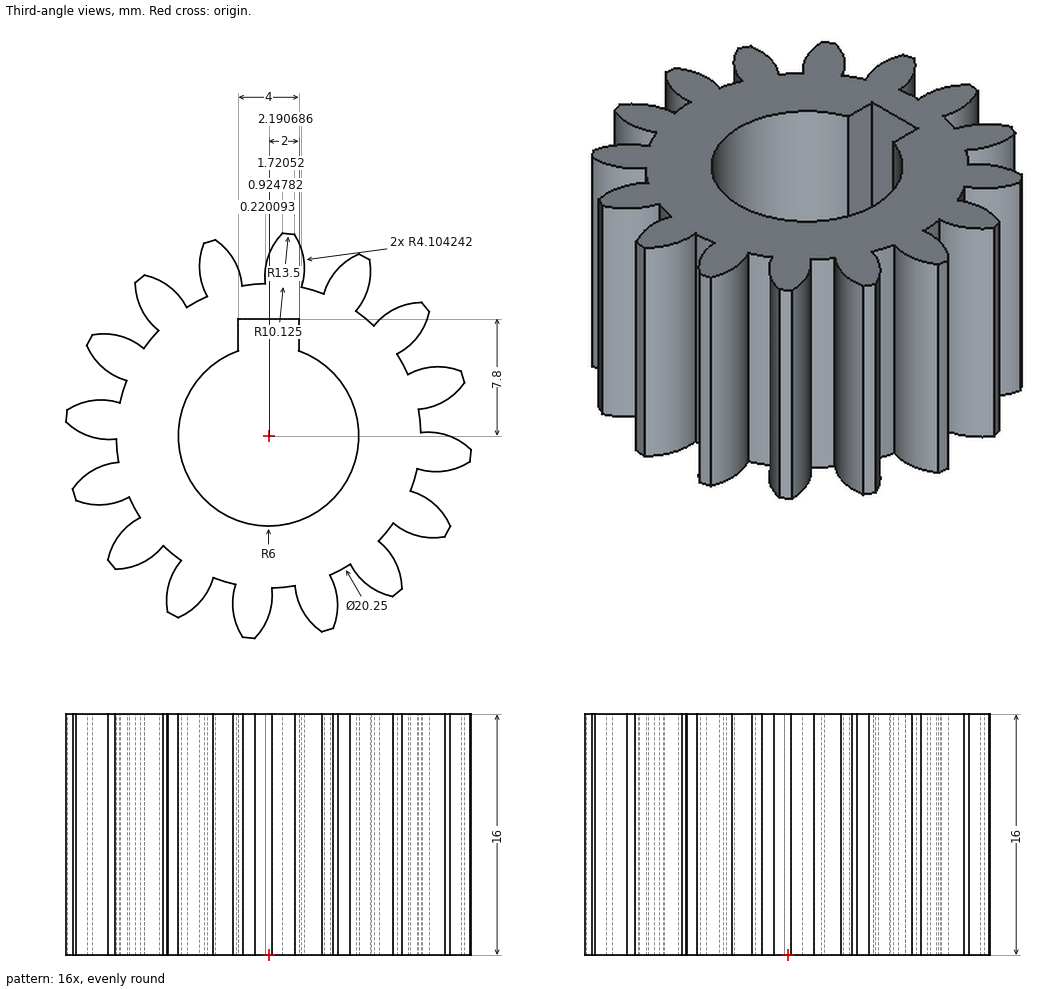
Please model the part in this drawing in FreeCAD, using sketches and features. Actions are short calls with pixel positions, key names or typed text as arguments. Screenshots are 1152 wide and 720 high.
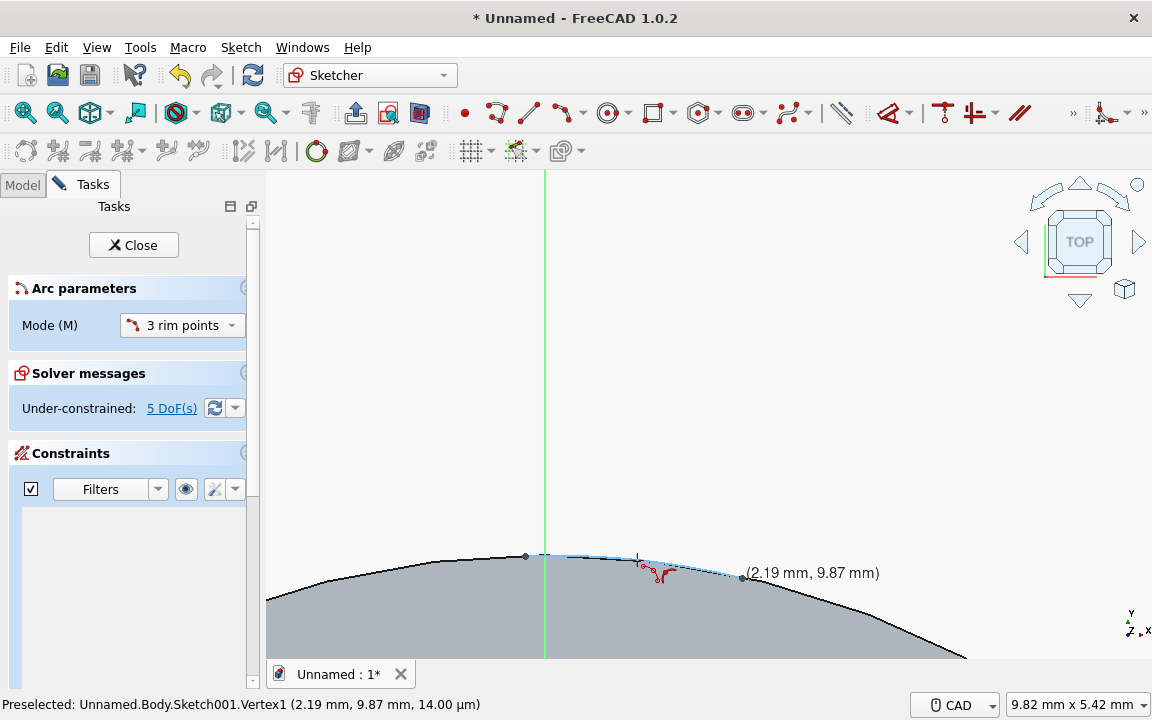
click(700, 261)
click(757, 414)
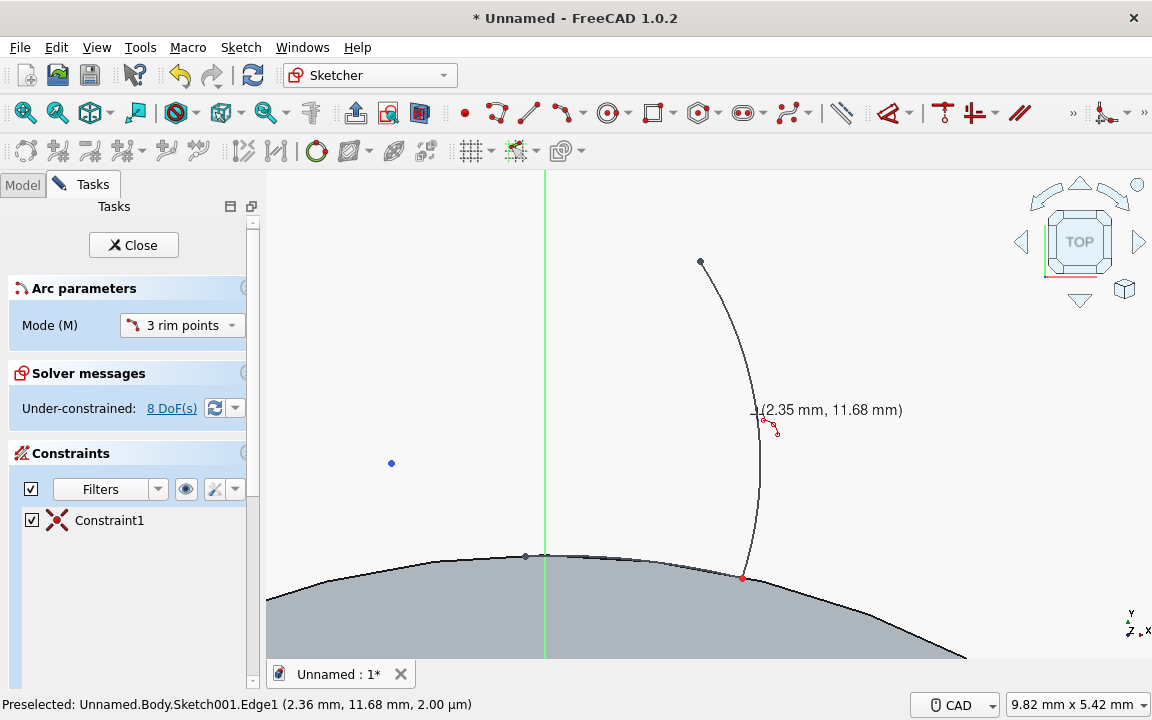
click(700, 262)
click(628, 254)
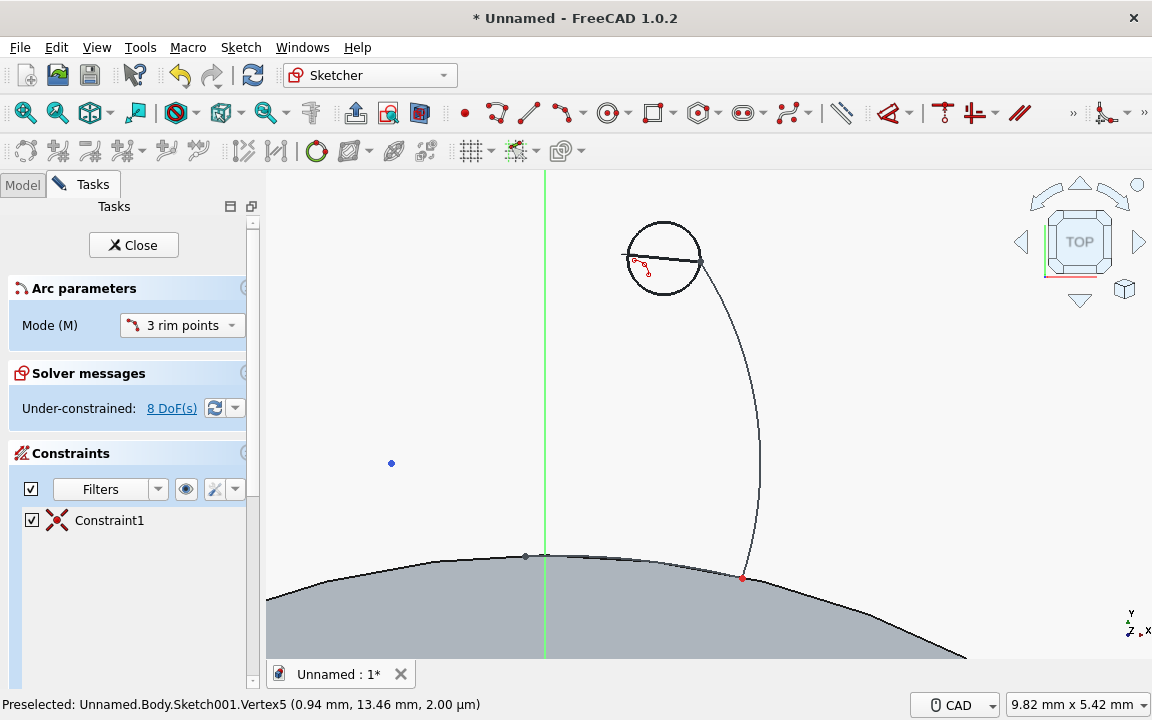
scroll(664, 257, up, 17)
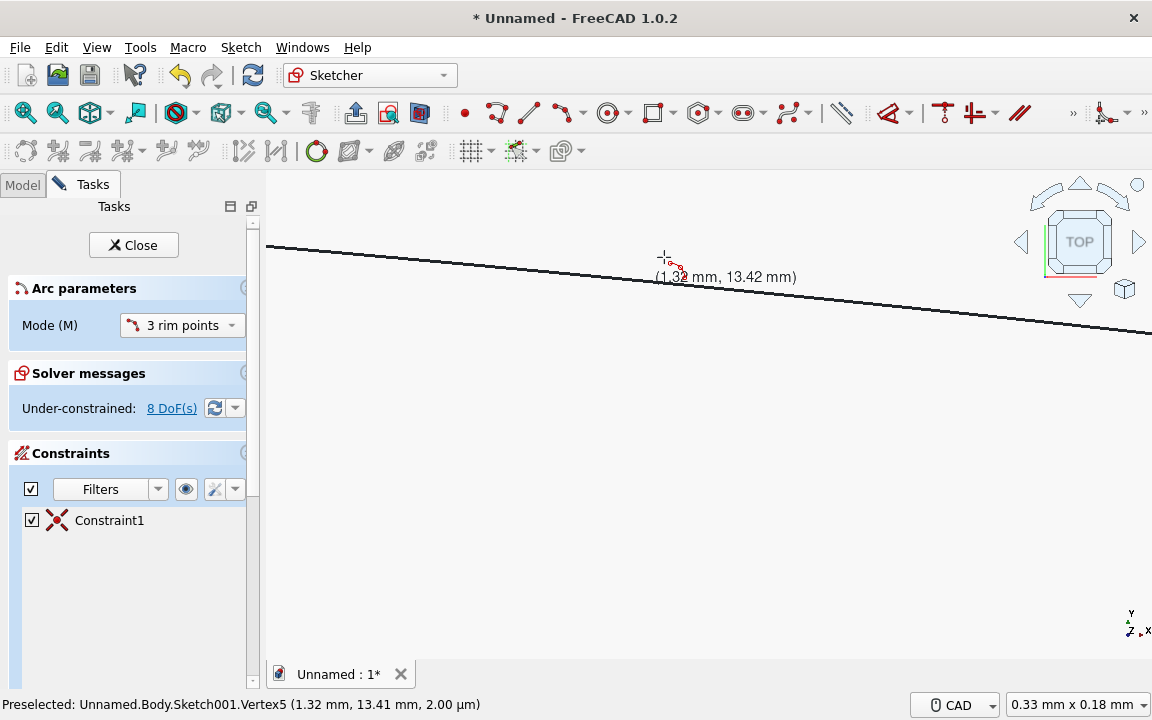
click(652, 242)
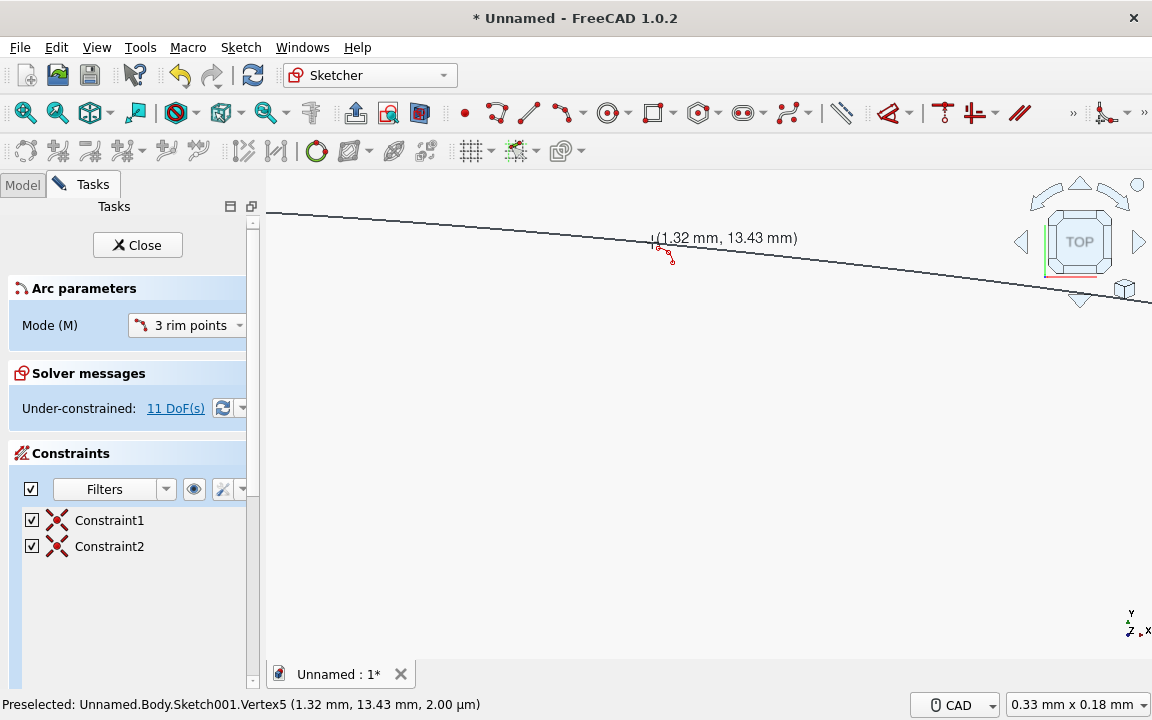
scroll(664, 256, down, 17)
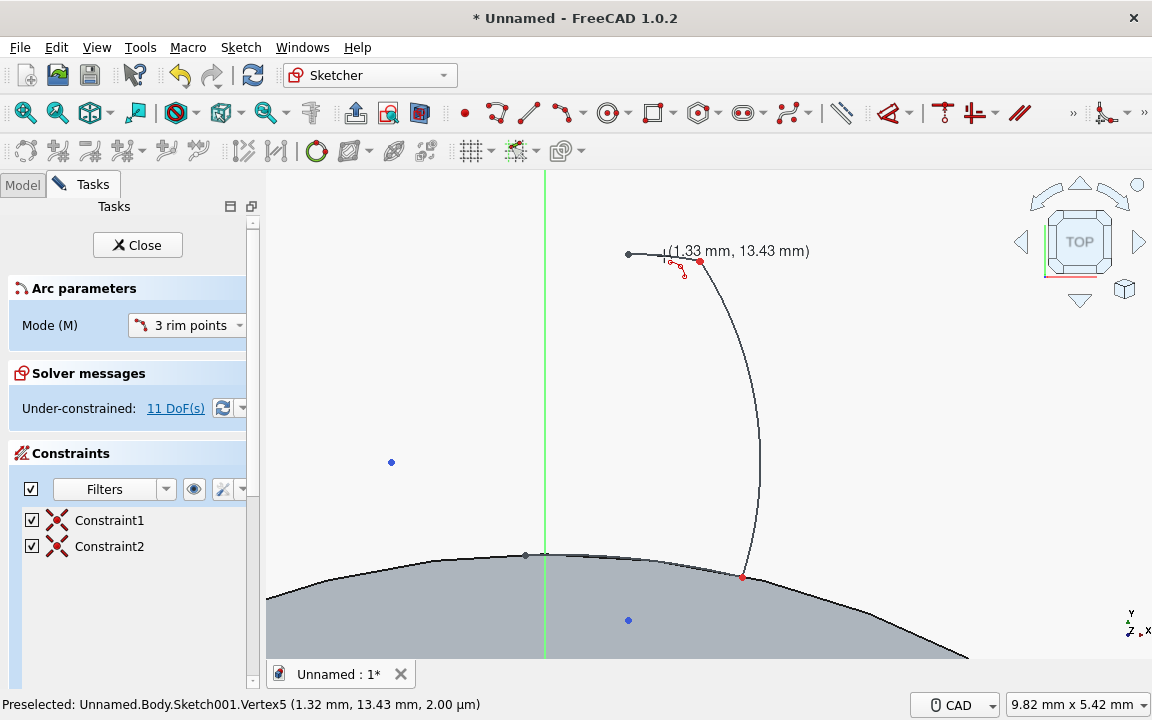
click(628, 254)
click(525, 555)
click(569, 332)
key(Escape)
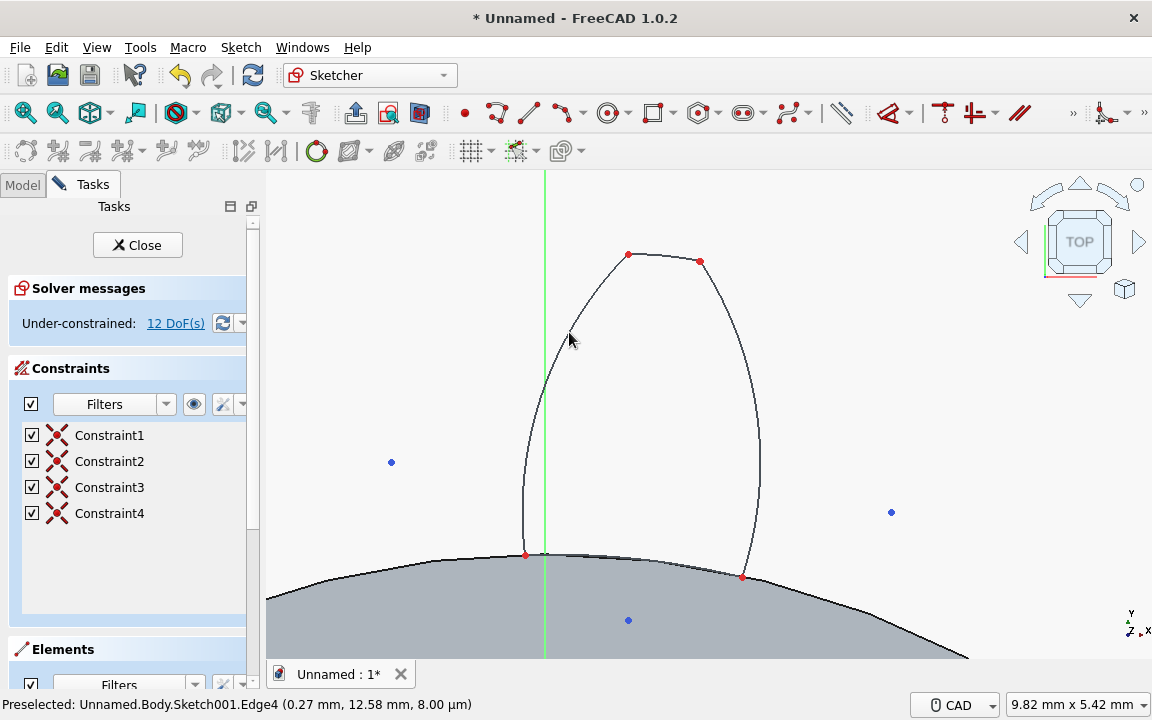
click(678, 564)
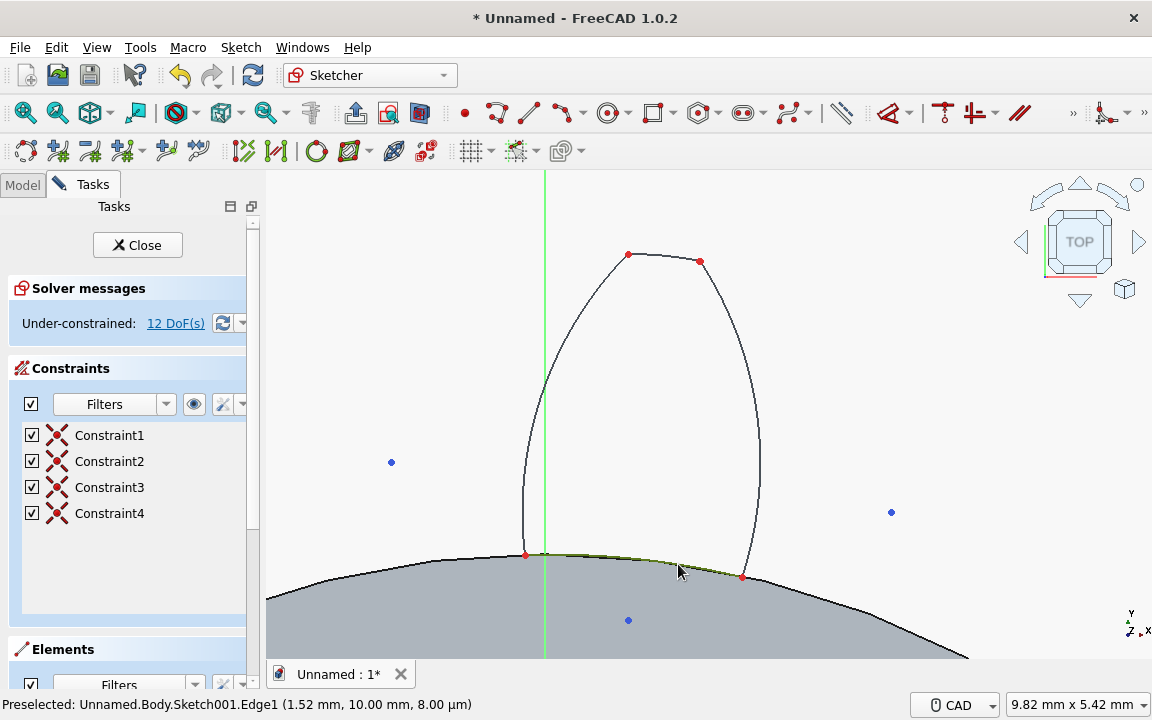
click(679, 257)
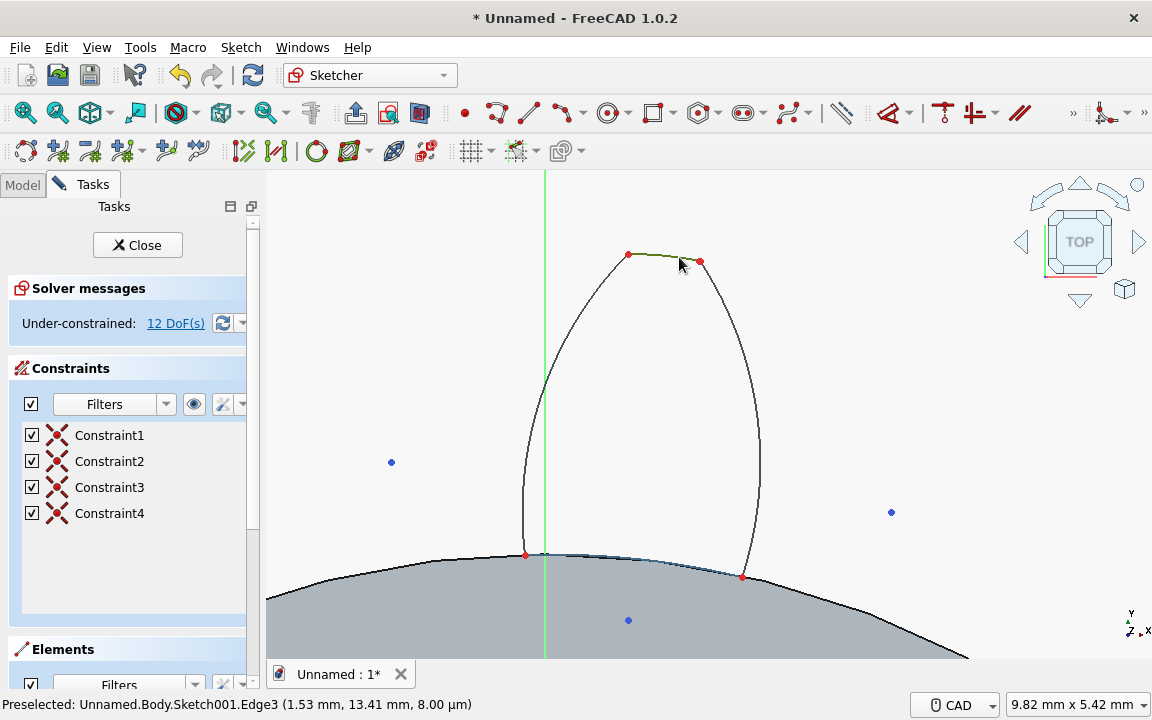
click(944, 114)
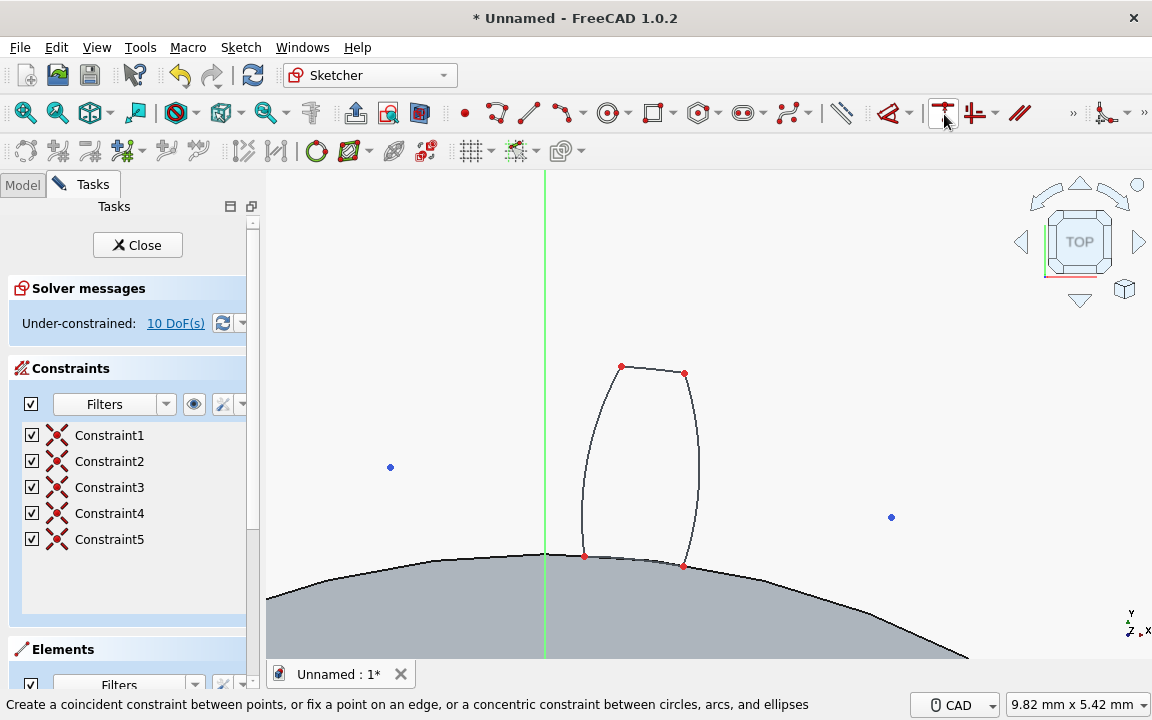
scroll(640, 258, down, 6)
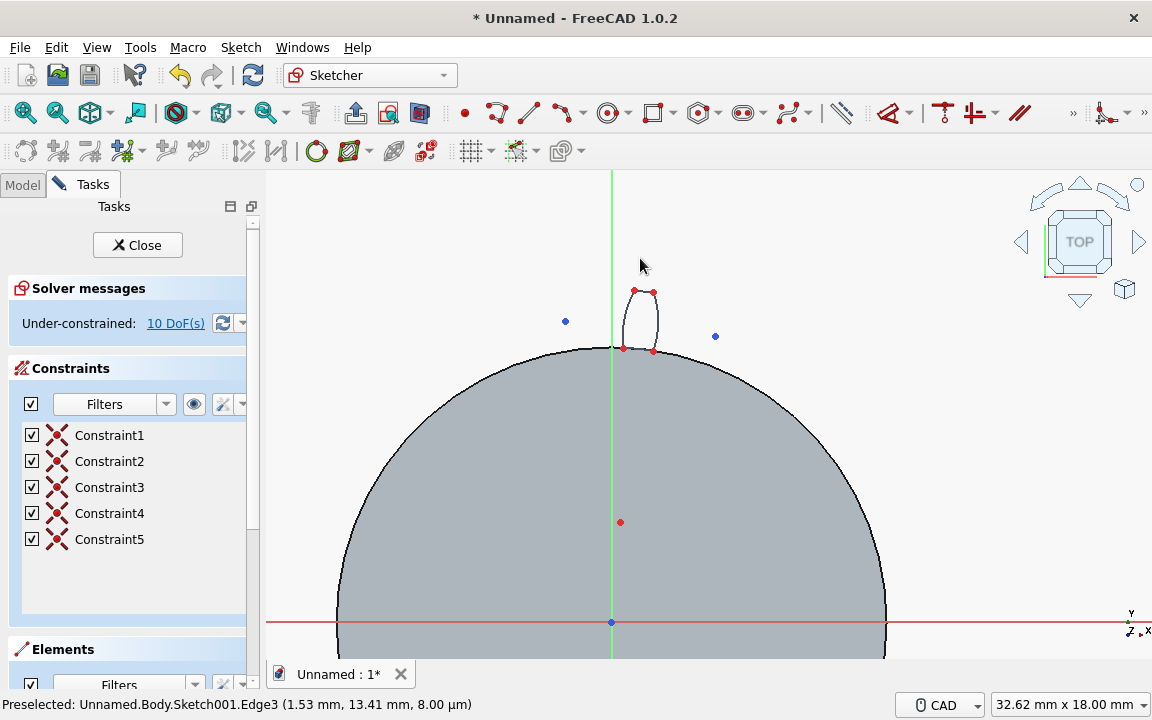
drag(602, 512, 631, 632)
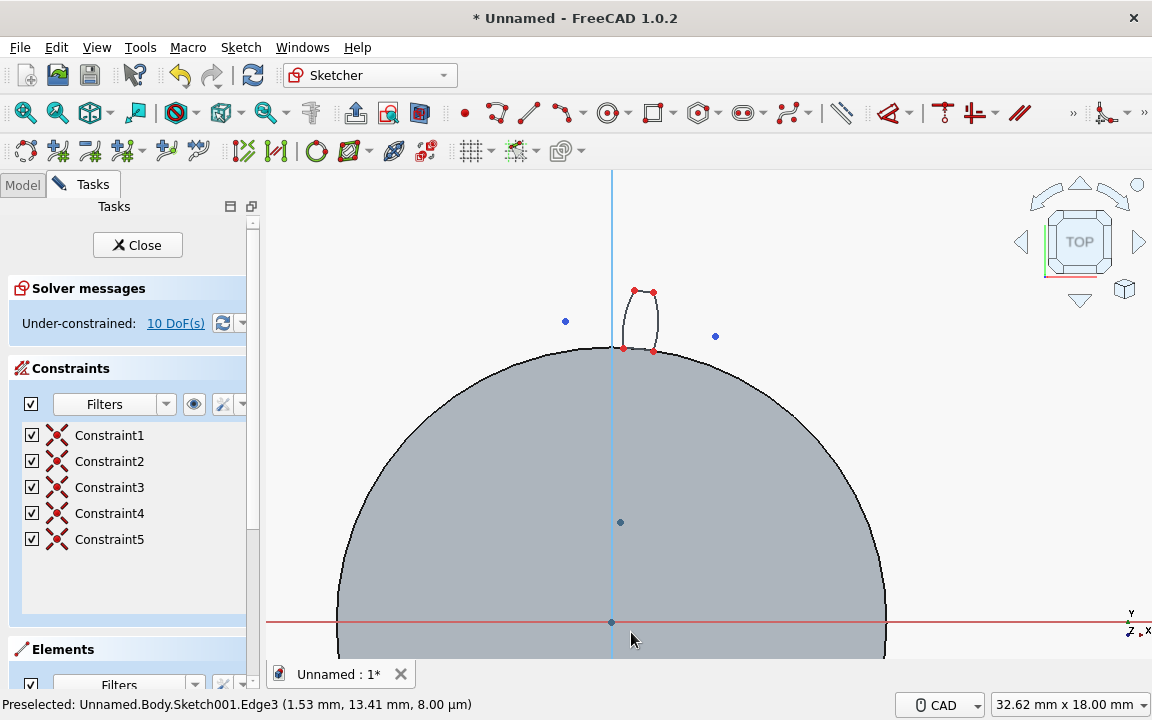
click(944, 114)